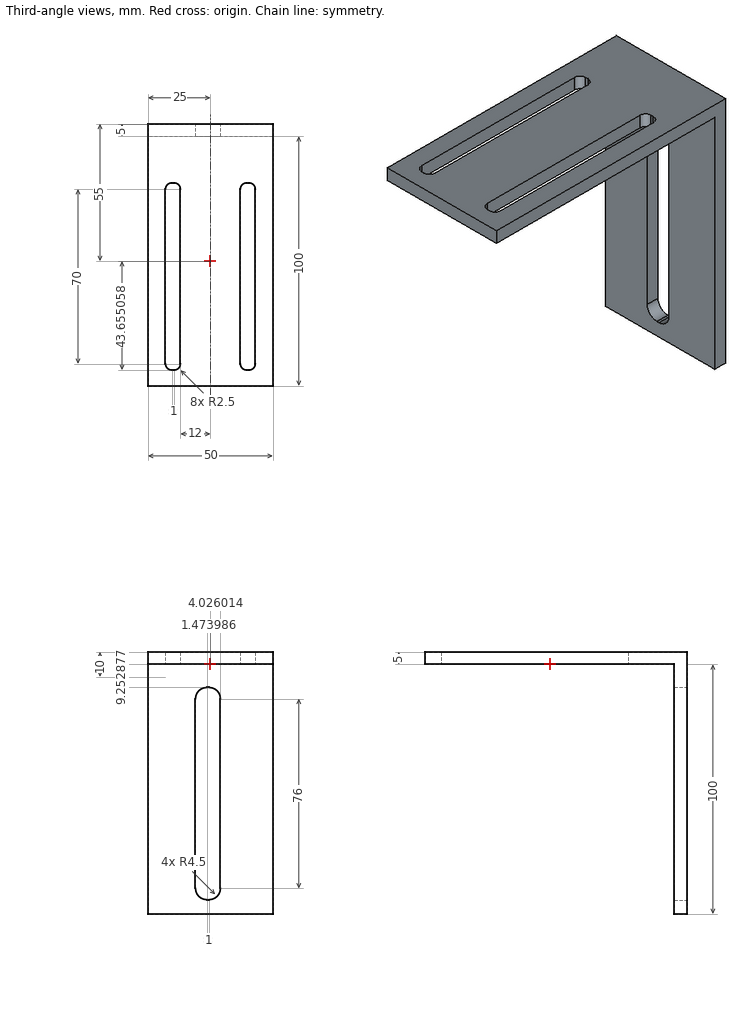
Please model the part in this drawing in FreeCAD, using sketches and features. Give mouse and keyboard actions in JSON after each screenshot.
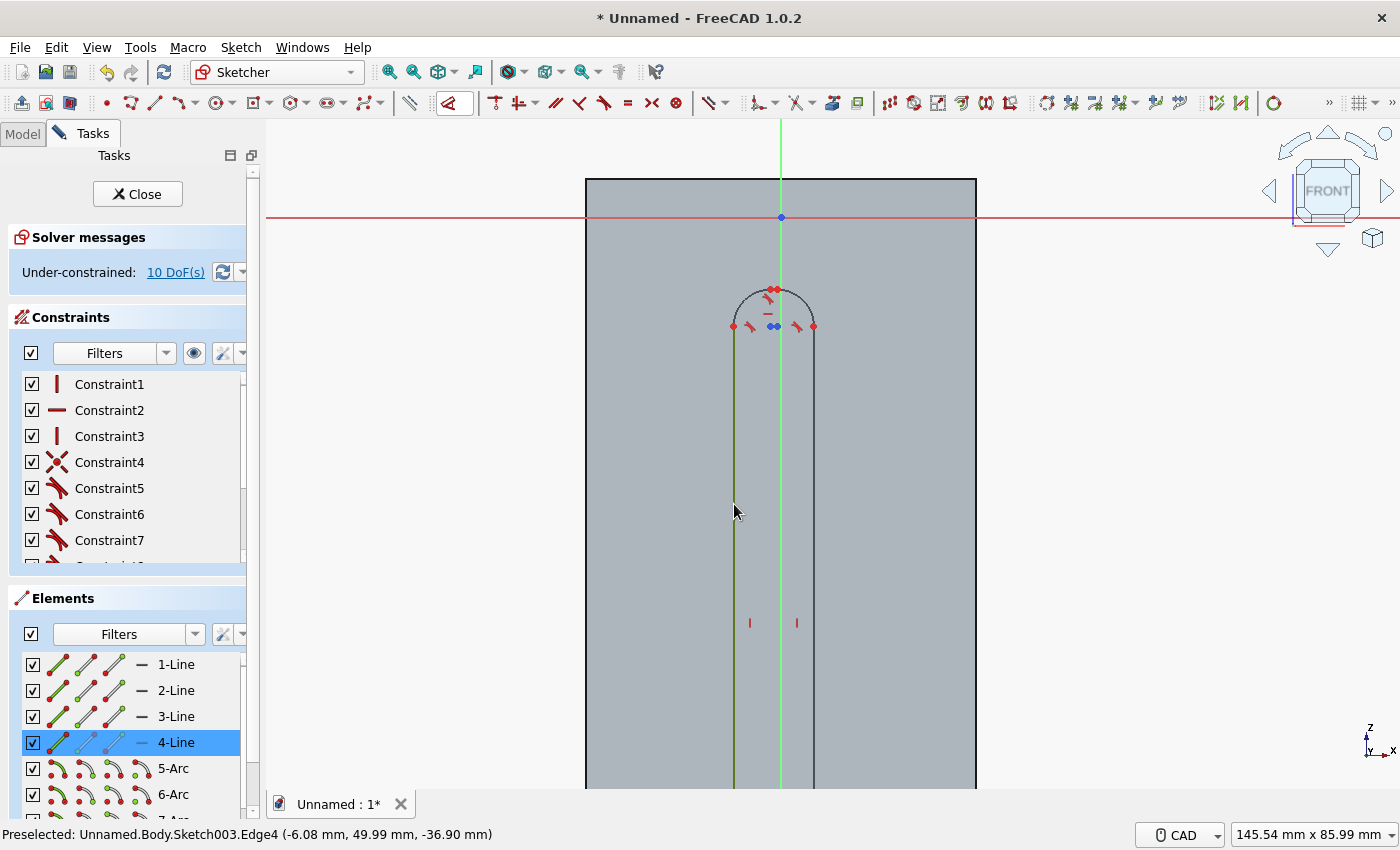
{"action": "scroll", "coordinate": [754, 295], "scroll_direction": "down", "scroll_amount": 3}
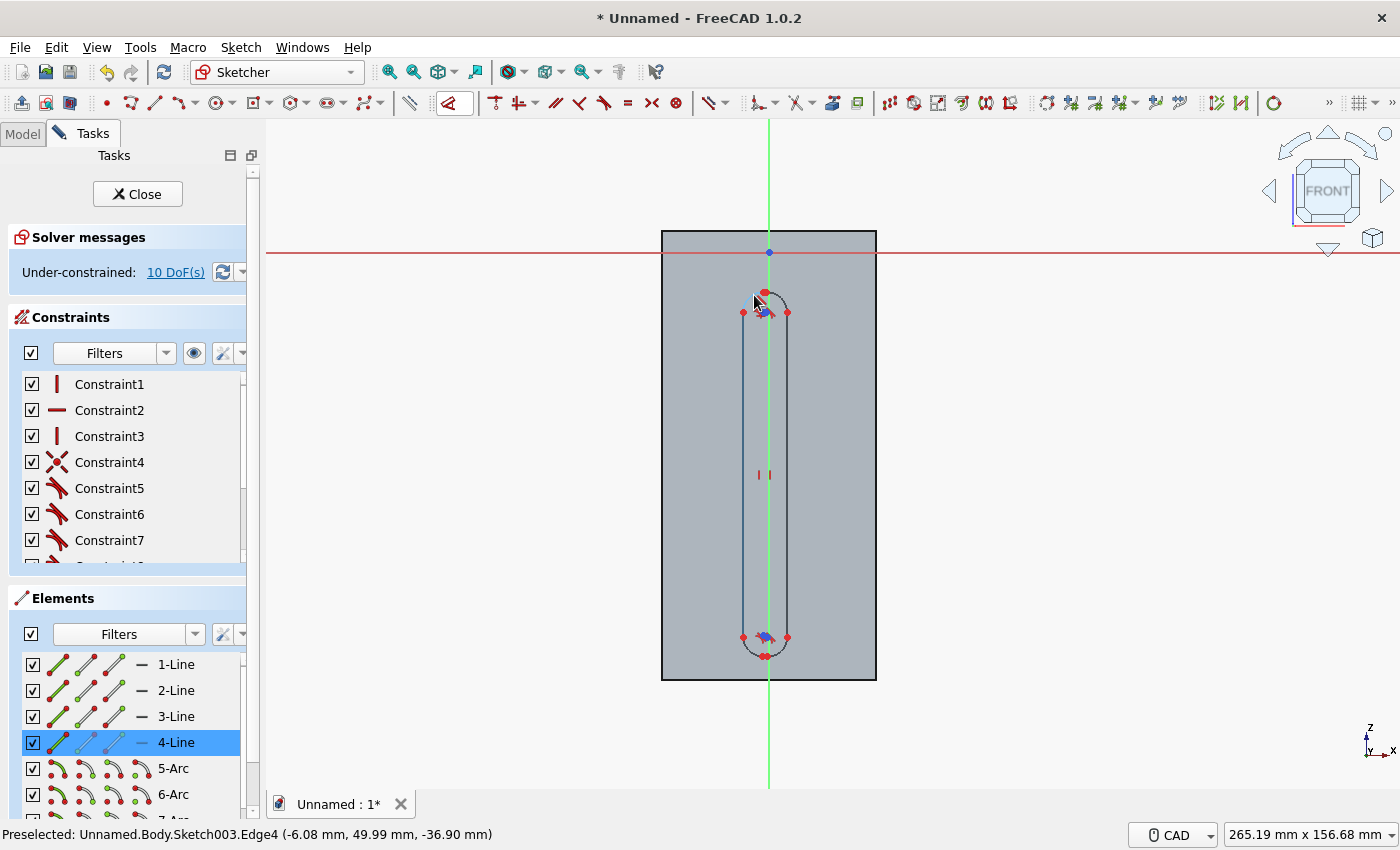
{"action": "scroll", "coordinate": [746, 646], "scroll_direction": "up", "scroll_amount": 3}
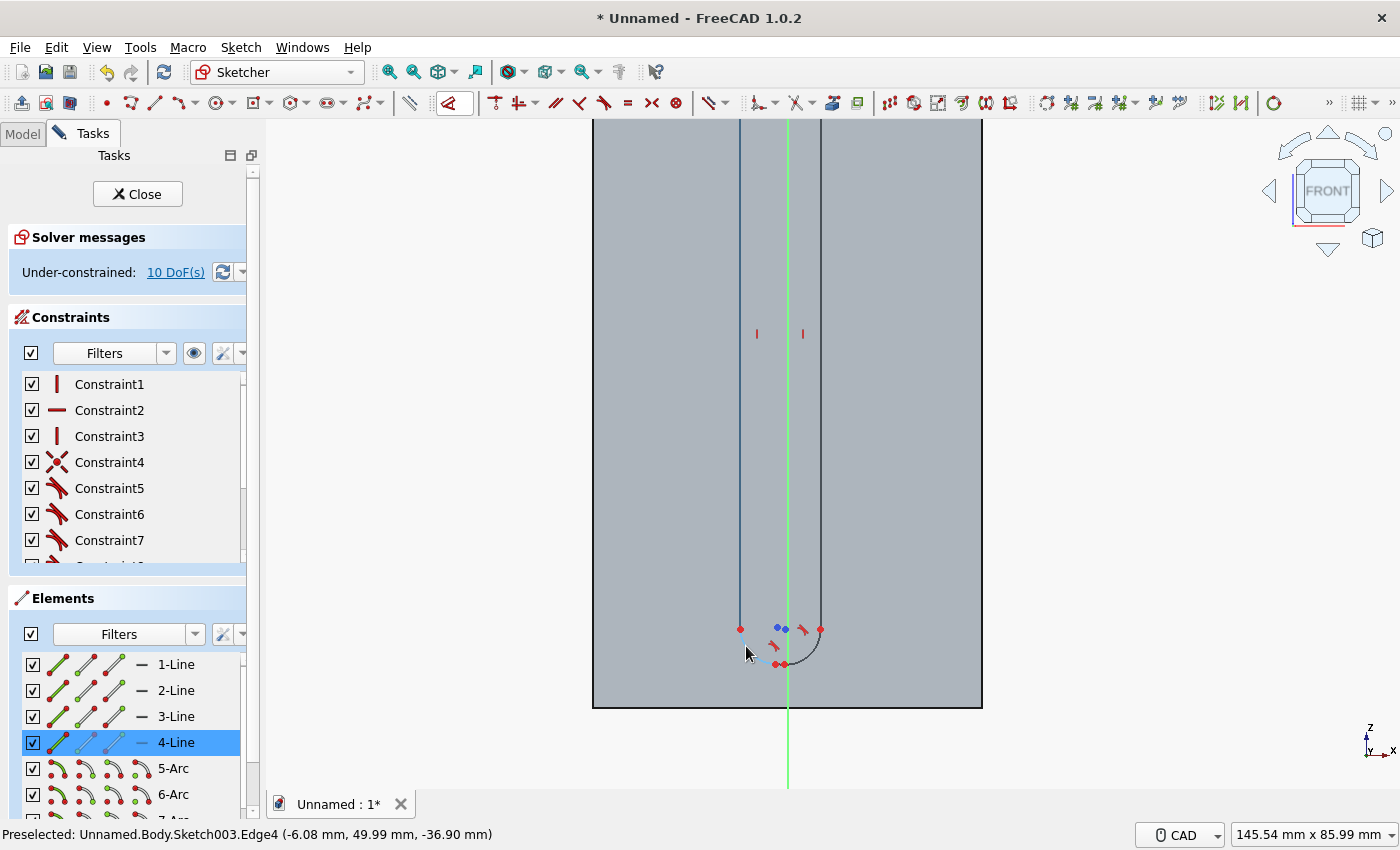
{"action": "left_click", "coordinate": [745, 645]}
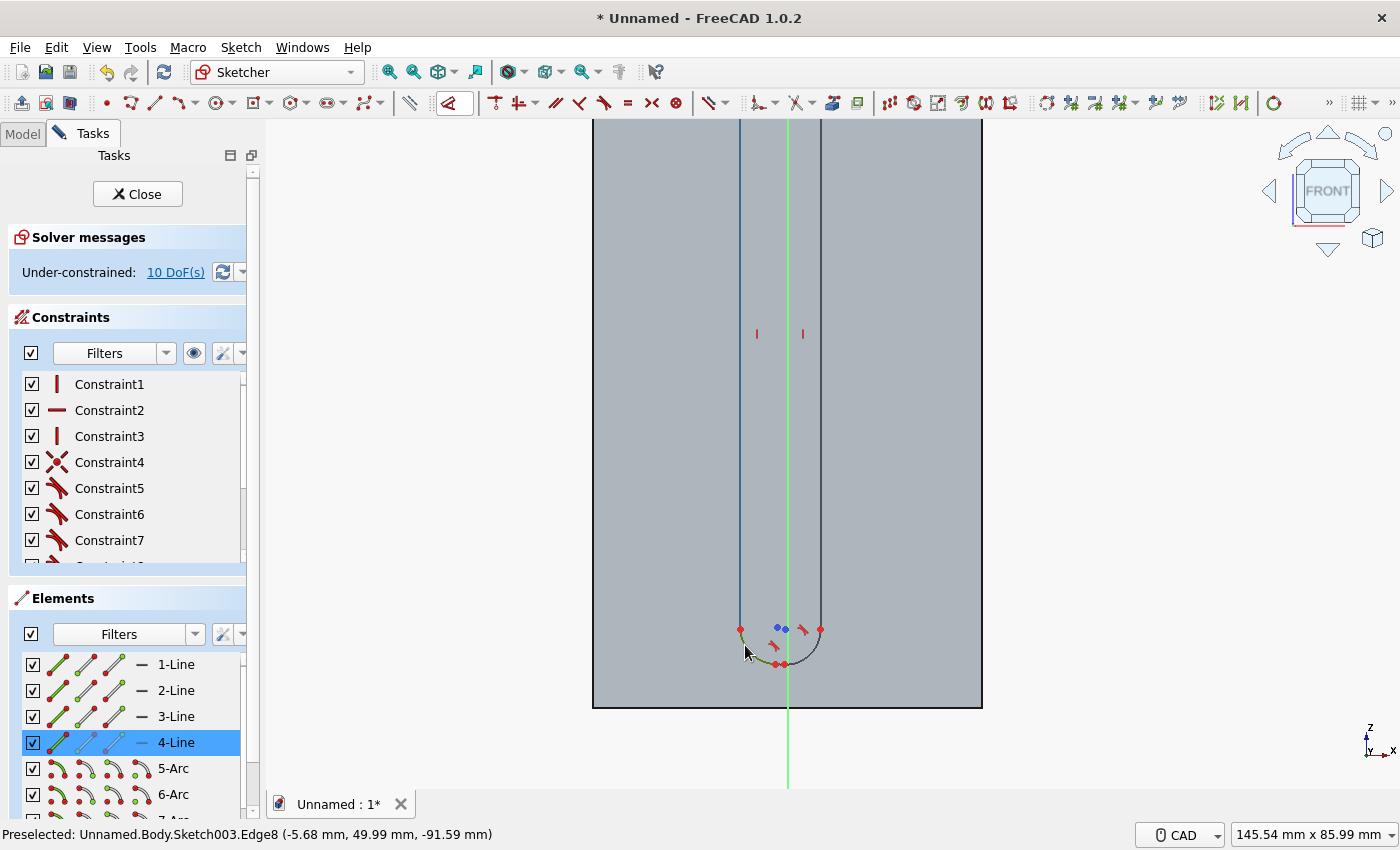
{"action": "key", "text": "t"}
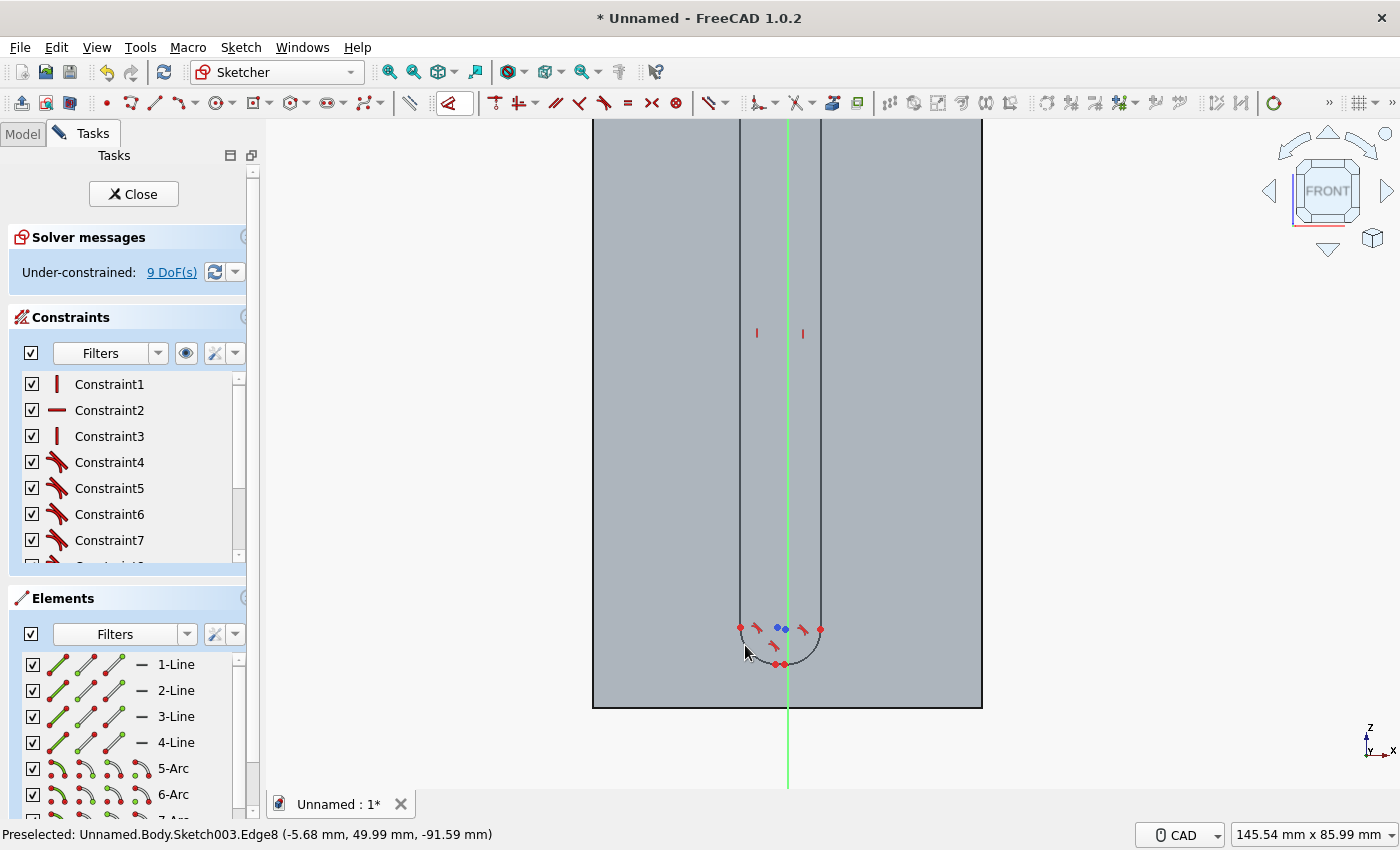
{"action": "left_click", "coordinate": [801, 661]}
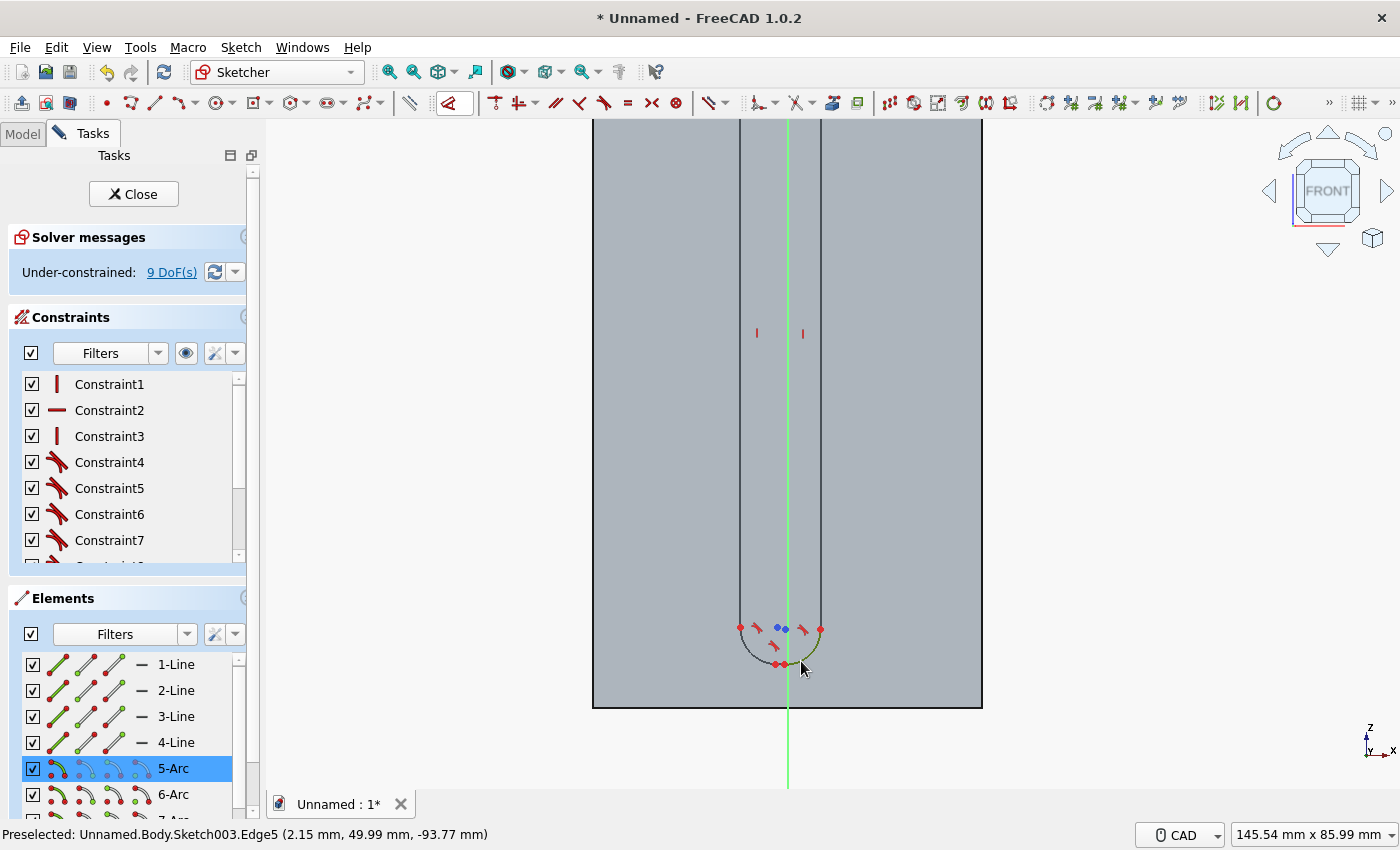
{"action": "scroll", "coordinate": [746, 647], "scroll_direction": "down", "scroll_amount": 3}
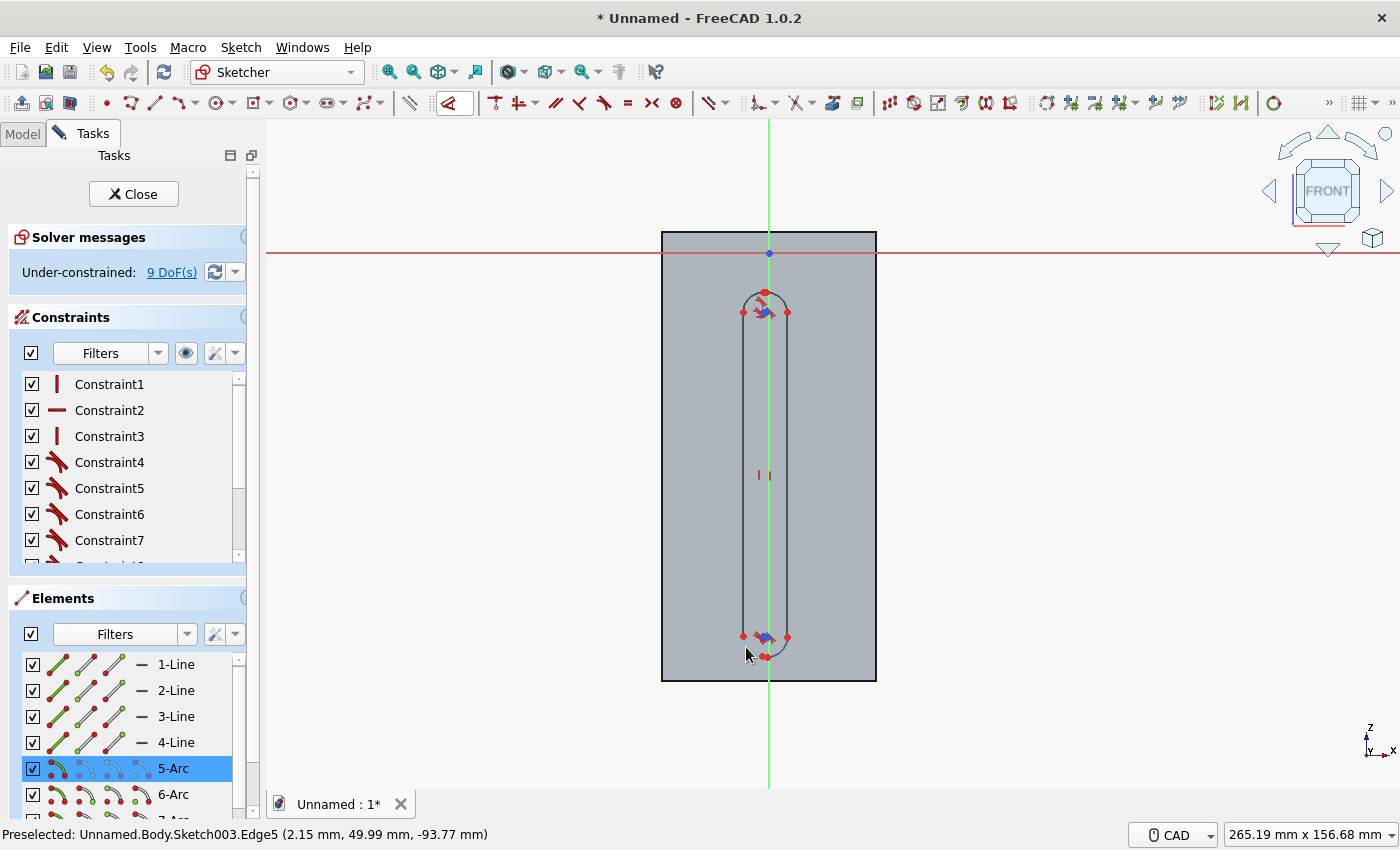
{"action": "scroll", "coordinate": [785, 304], "scroll_direction": "up", "scroll_amount": 2}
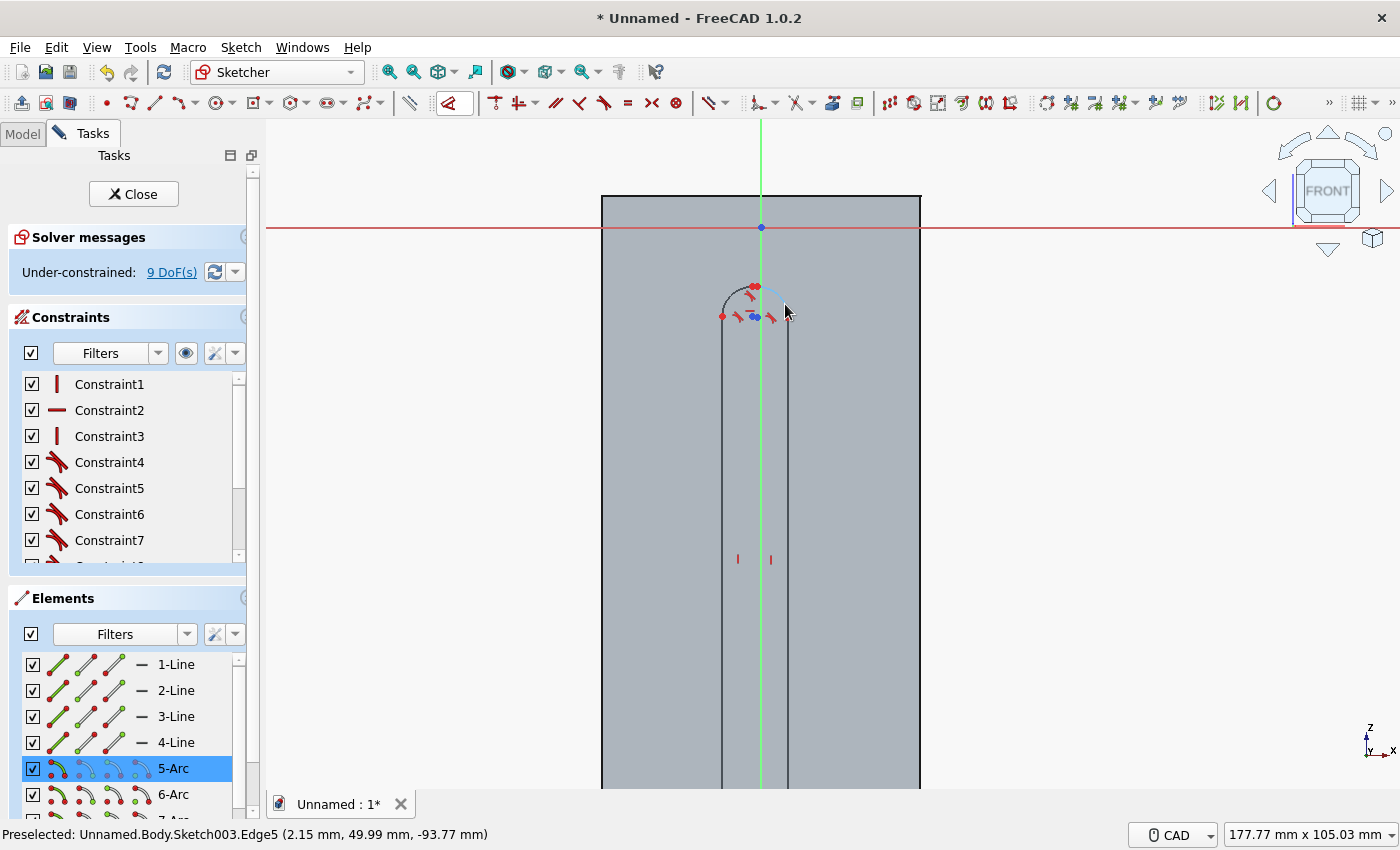
{"action": "left_click", "coordinate": [785, 303]}